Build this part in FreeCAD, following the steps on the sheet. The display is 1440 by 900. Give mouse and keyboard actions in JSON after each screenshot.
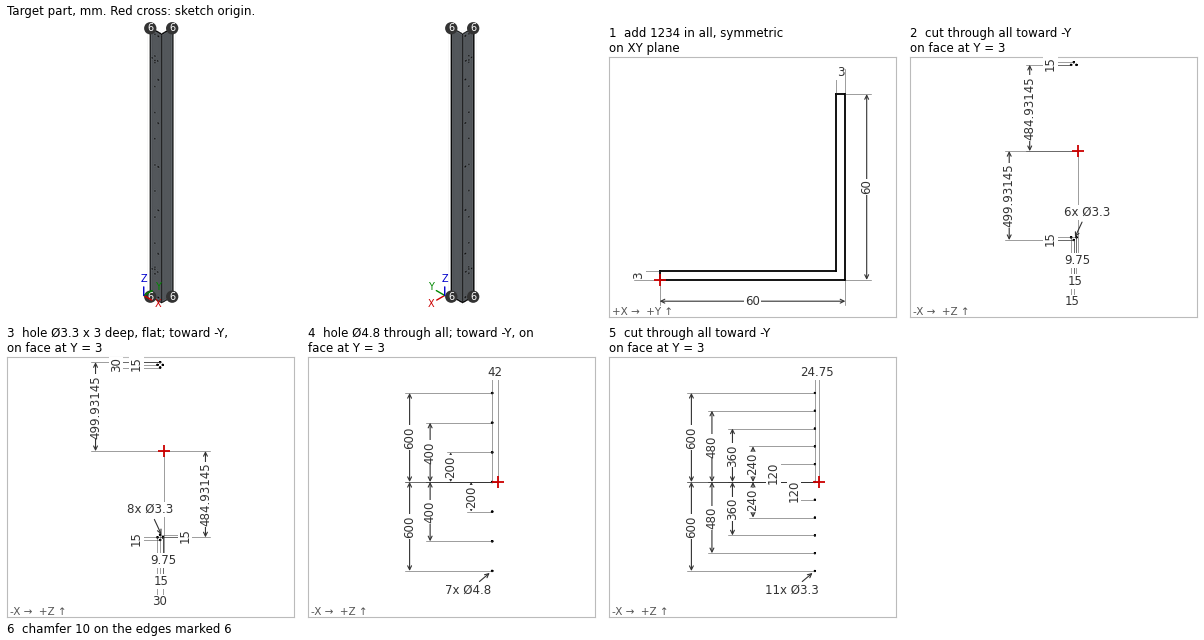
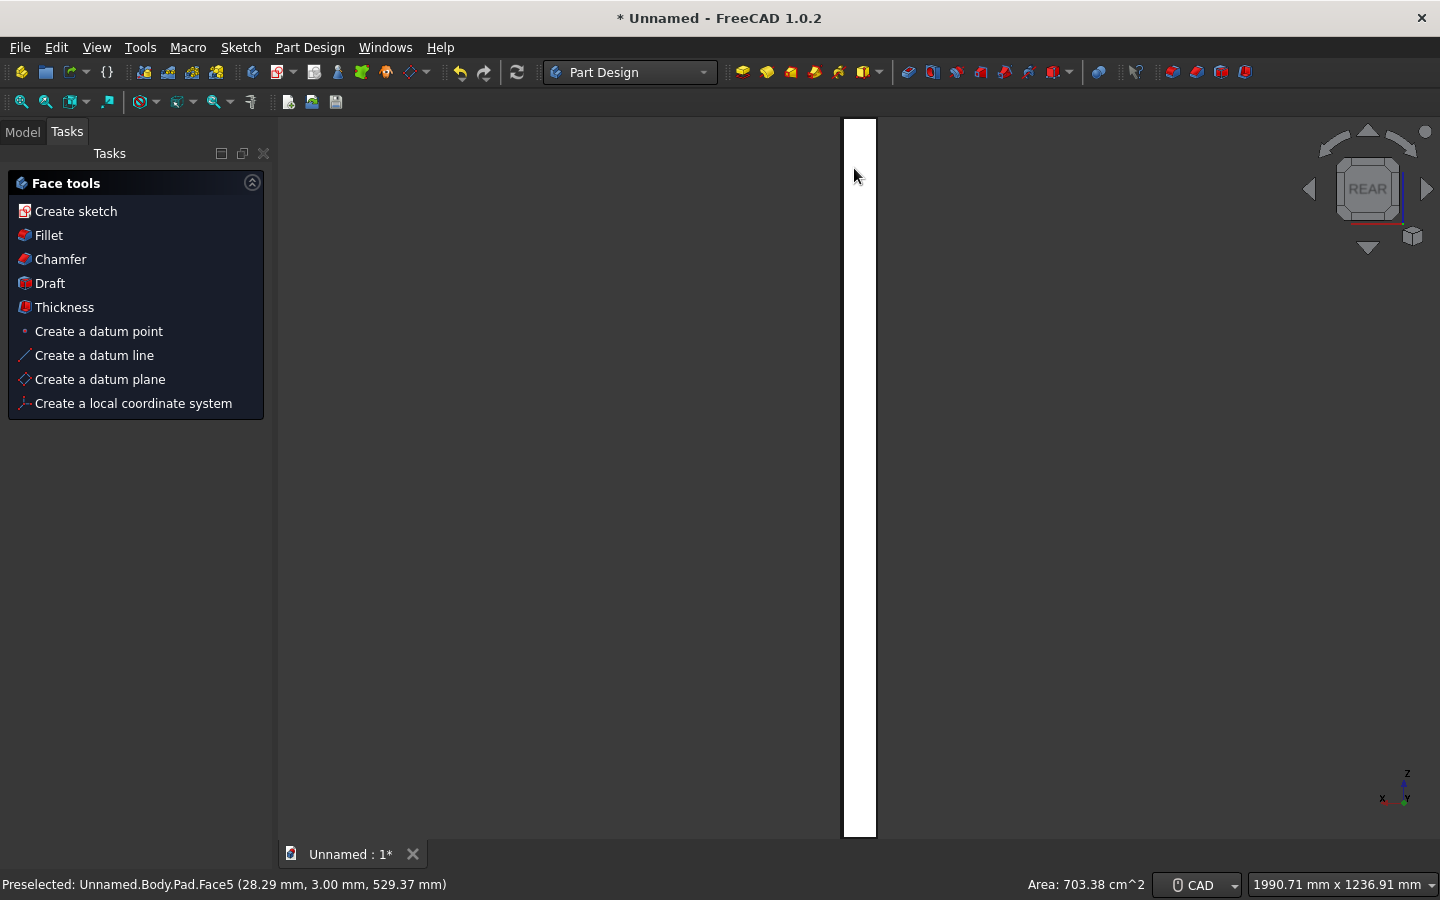
{"action": "left_click", "coordinate": [278, 72]}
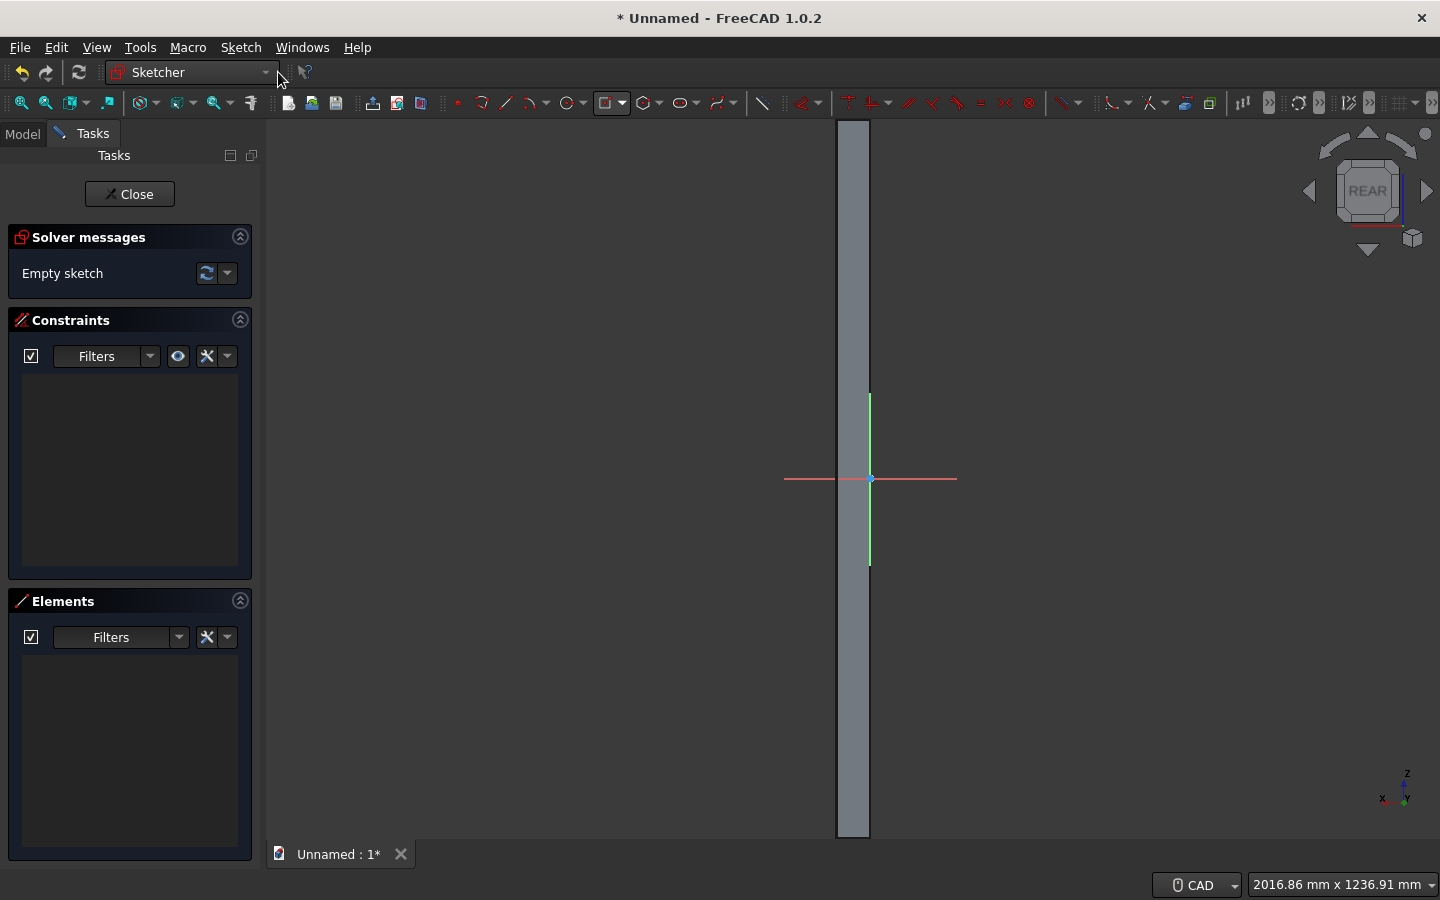
{"action": "left_click", "coordinate": [422, 104]}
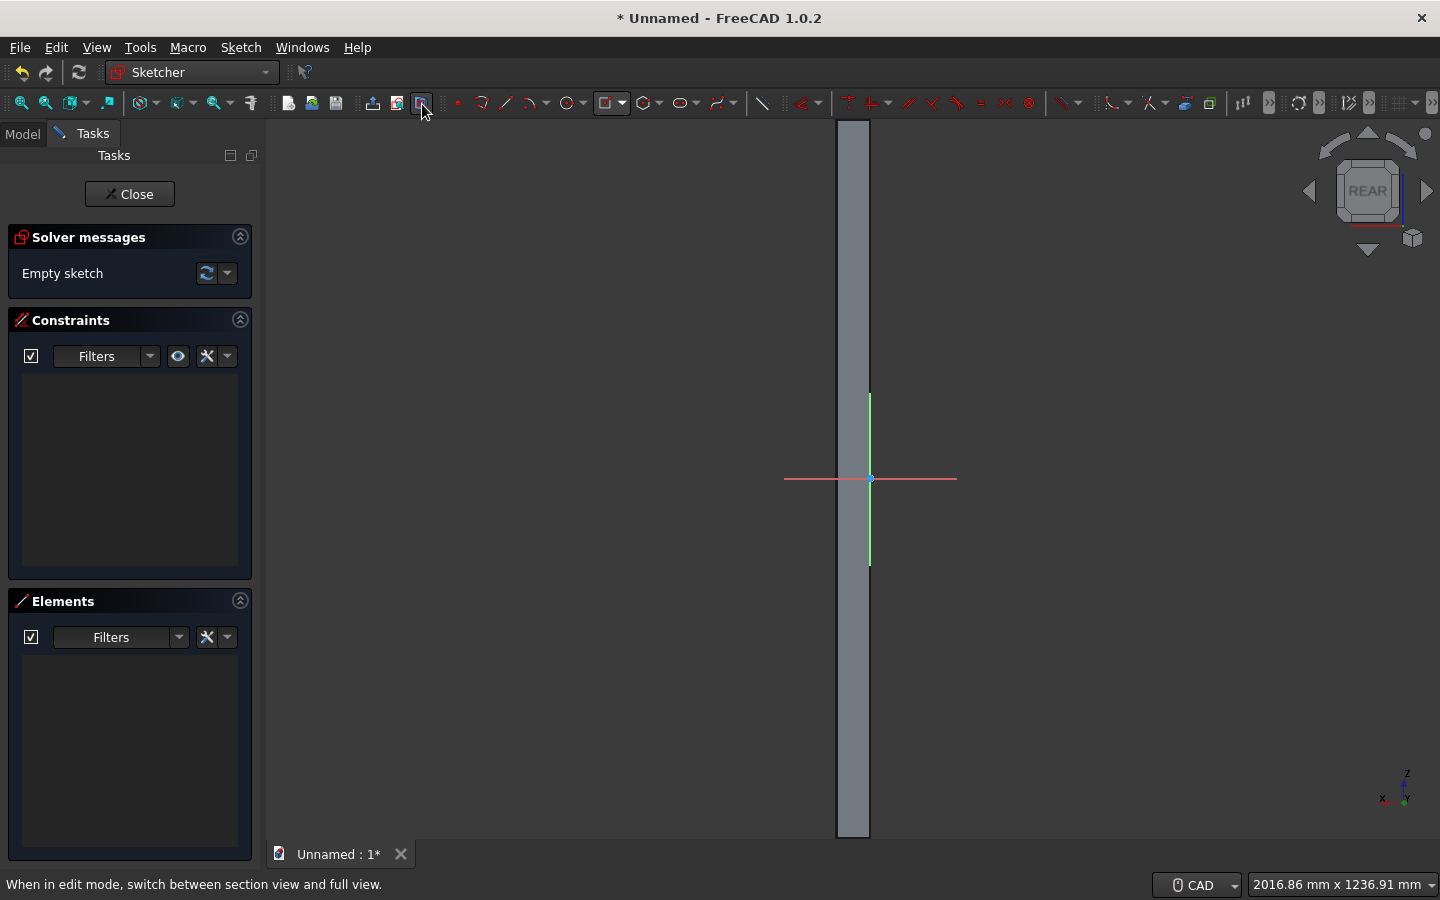
{"action": "left_click", "coordinate": [568, 104]}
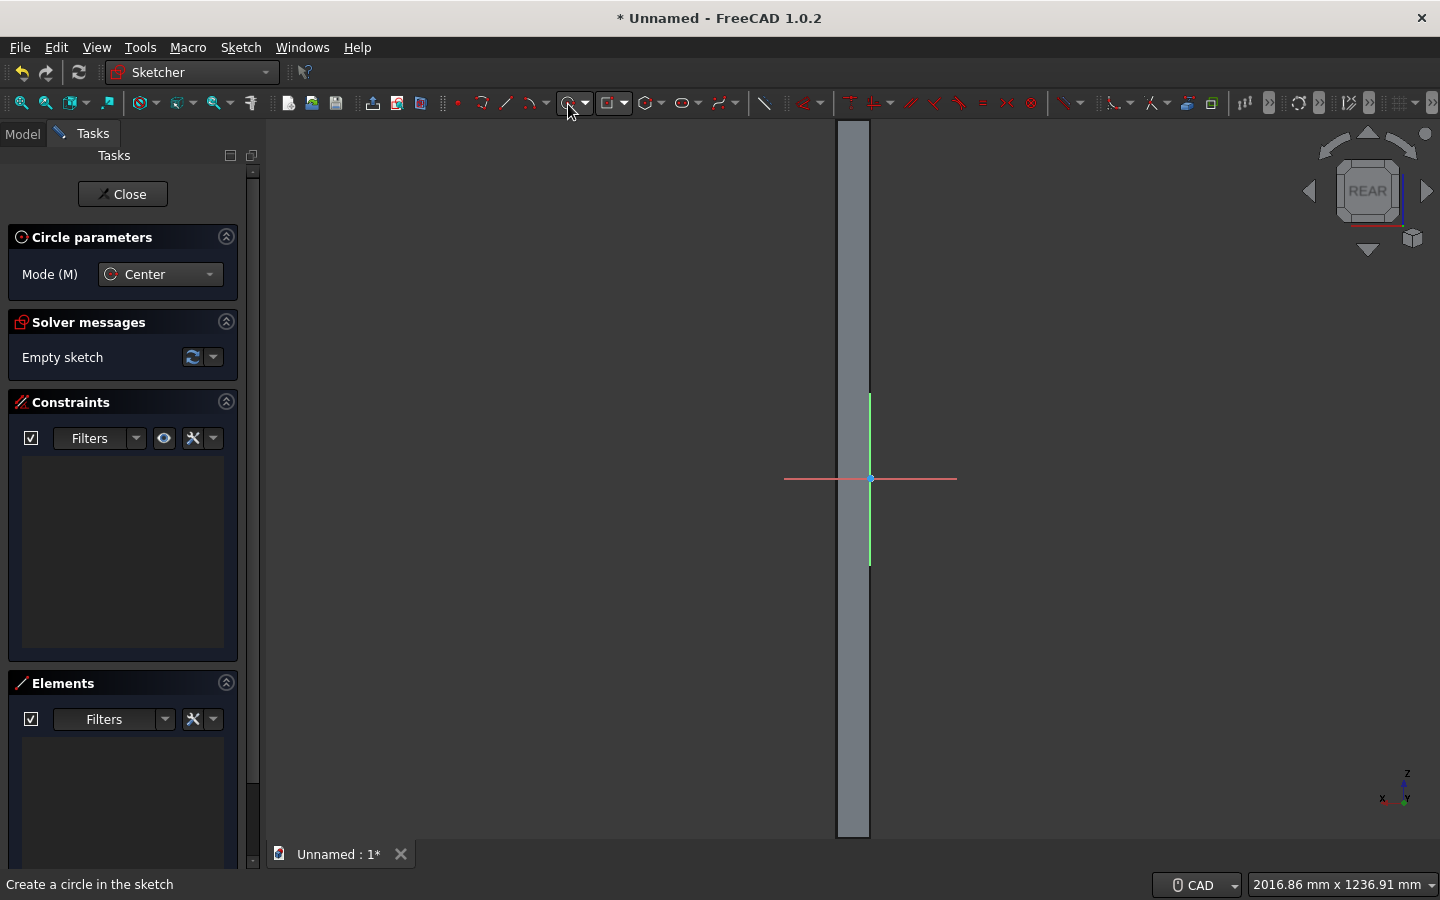
{"action": "scroll", "coordinate": [856, 770], "scroll_direction": "up", "scroll_amount": 16}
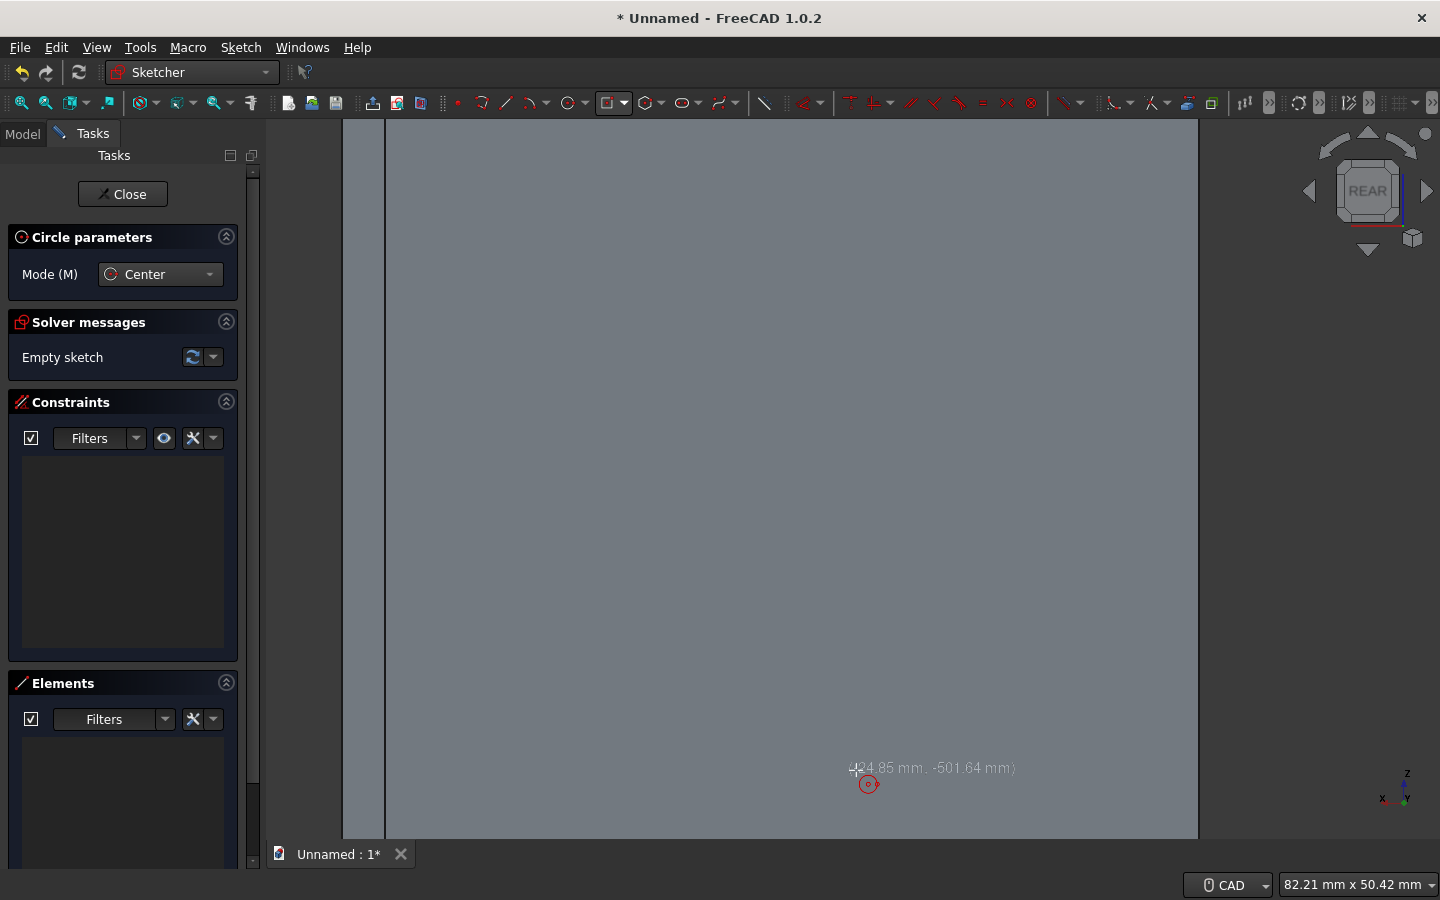
{"action": "scroll", "coordinate": [779, 771], "scroll_direction": "down", "scroll_amount": 16}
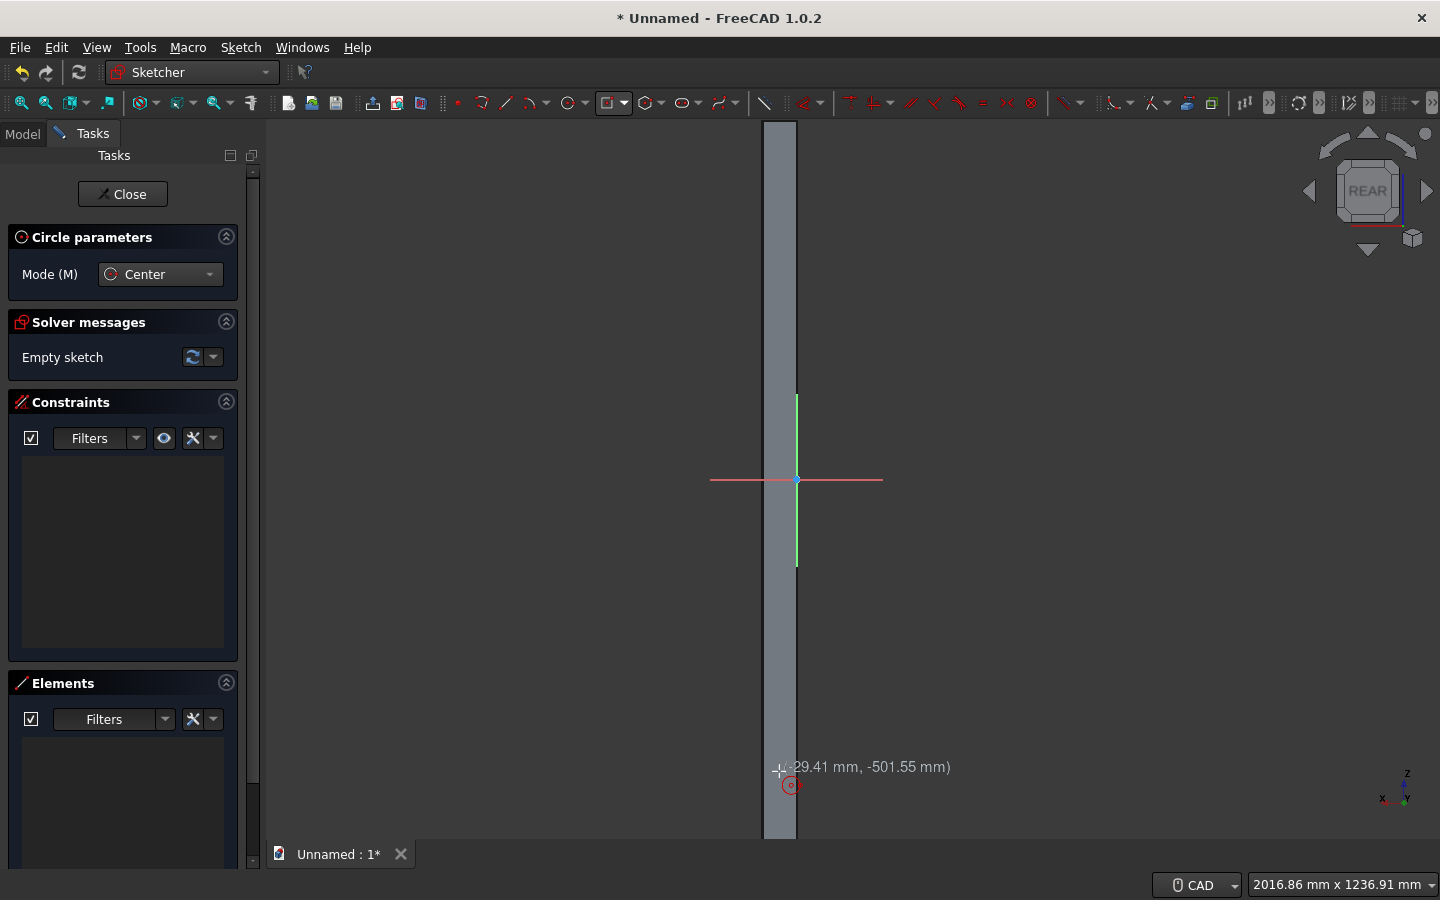
{"action": "left_click", "coordinate": [782, 771]}
{"action": "mouse_move", "coordinate": [781, 770]}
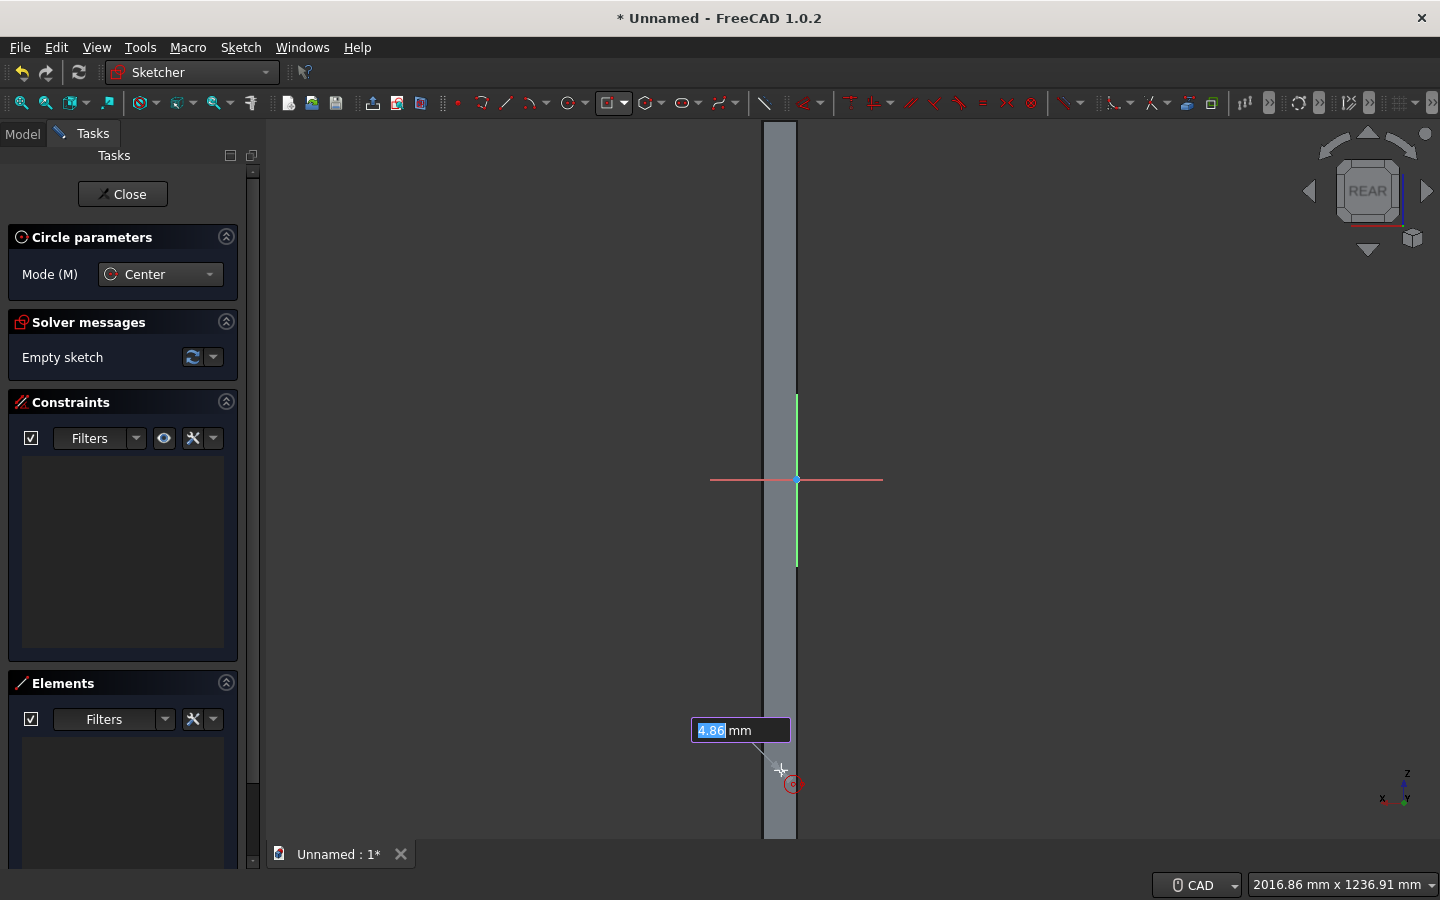
{"action": "type", "text": "3.3"}
{"action": "key", "text": "Return"}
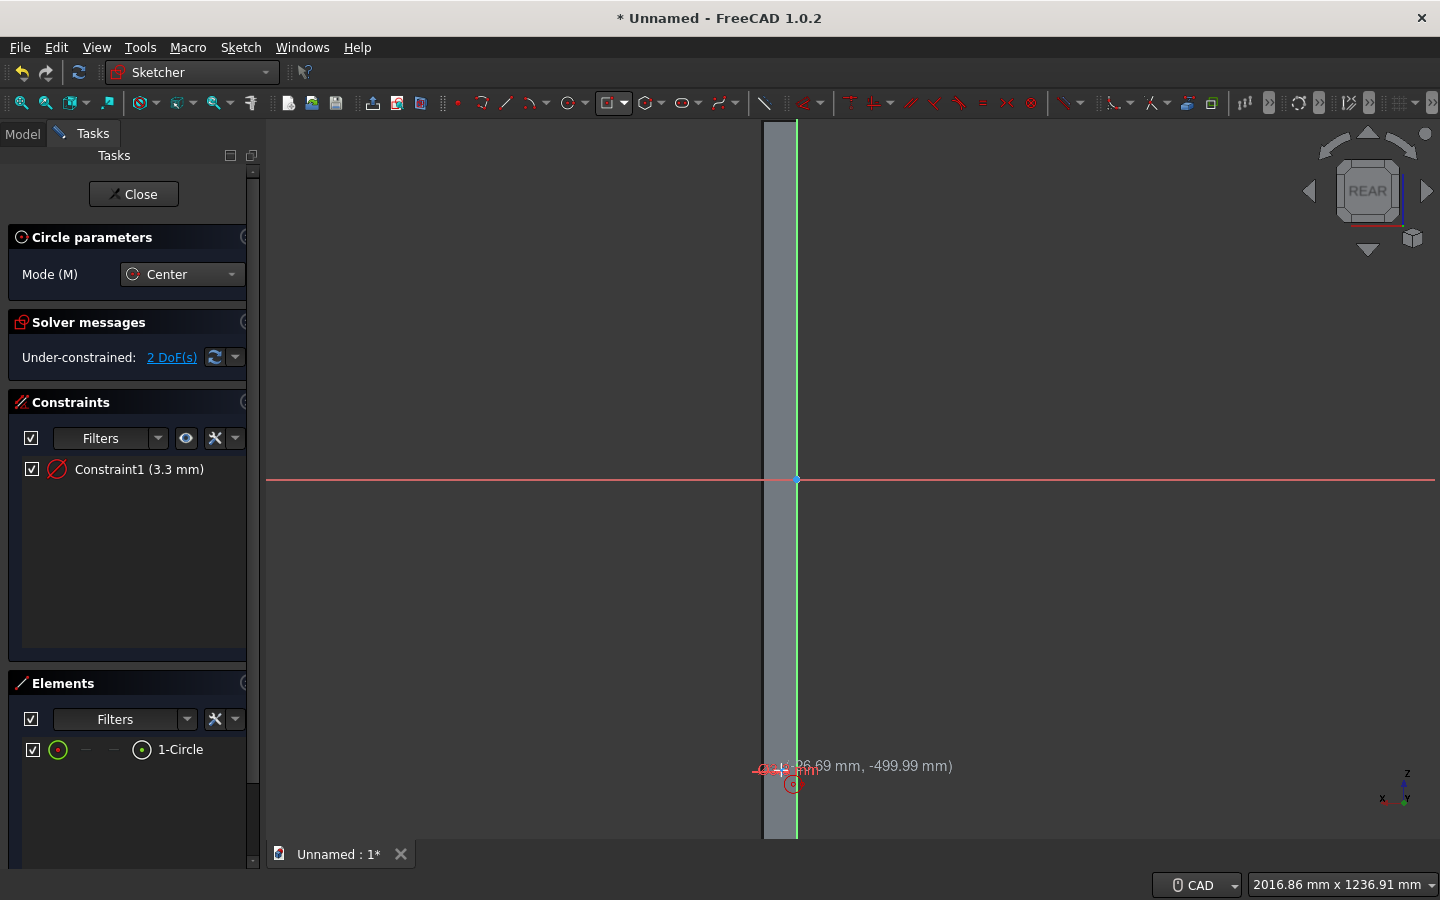
{"action": "scroll", "coordinate": [791, 762], "scroll_direction": "up", "scroll_amount": 16}